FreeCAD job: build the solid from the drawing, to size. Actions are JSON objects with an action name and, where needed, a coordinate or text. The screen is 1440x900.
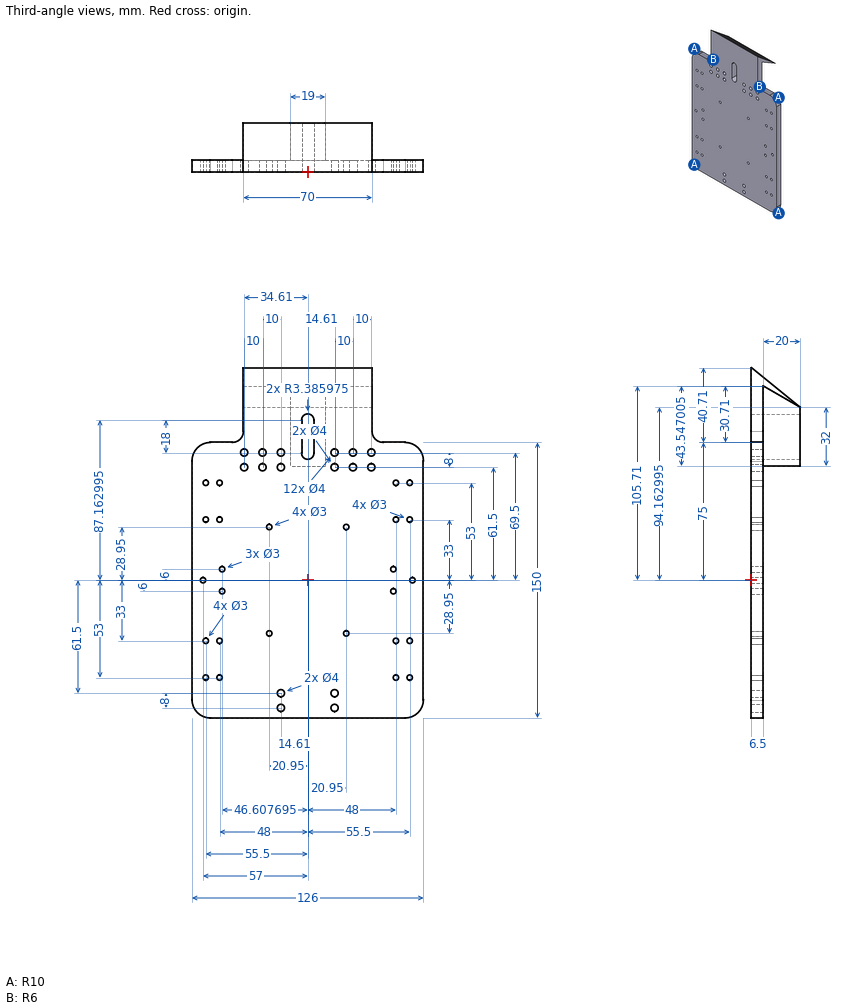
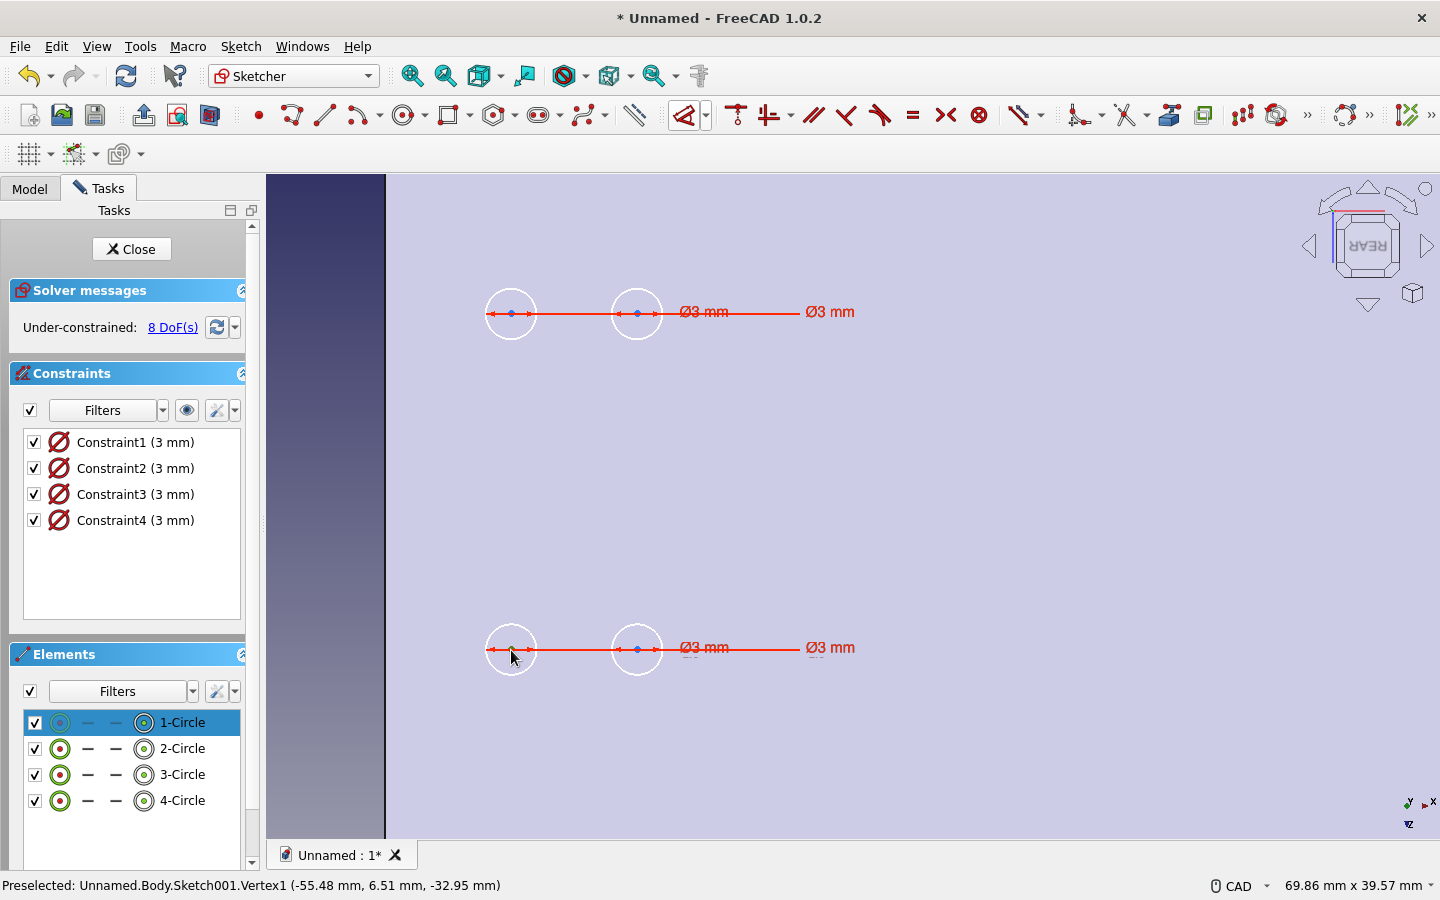
{"action": "left_click", "coordinate": [637, 650]}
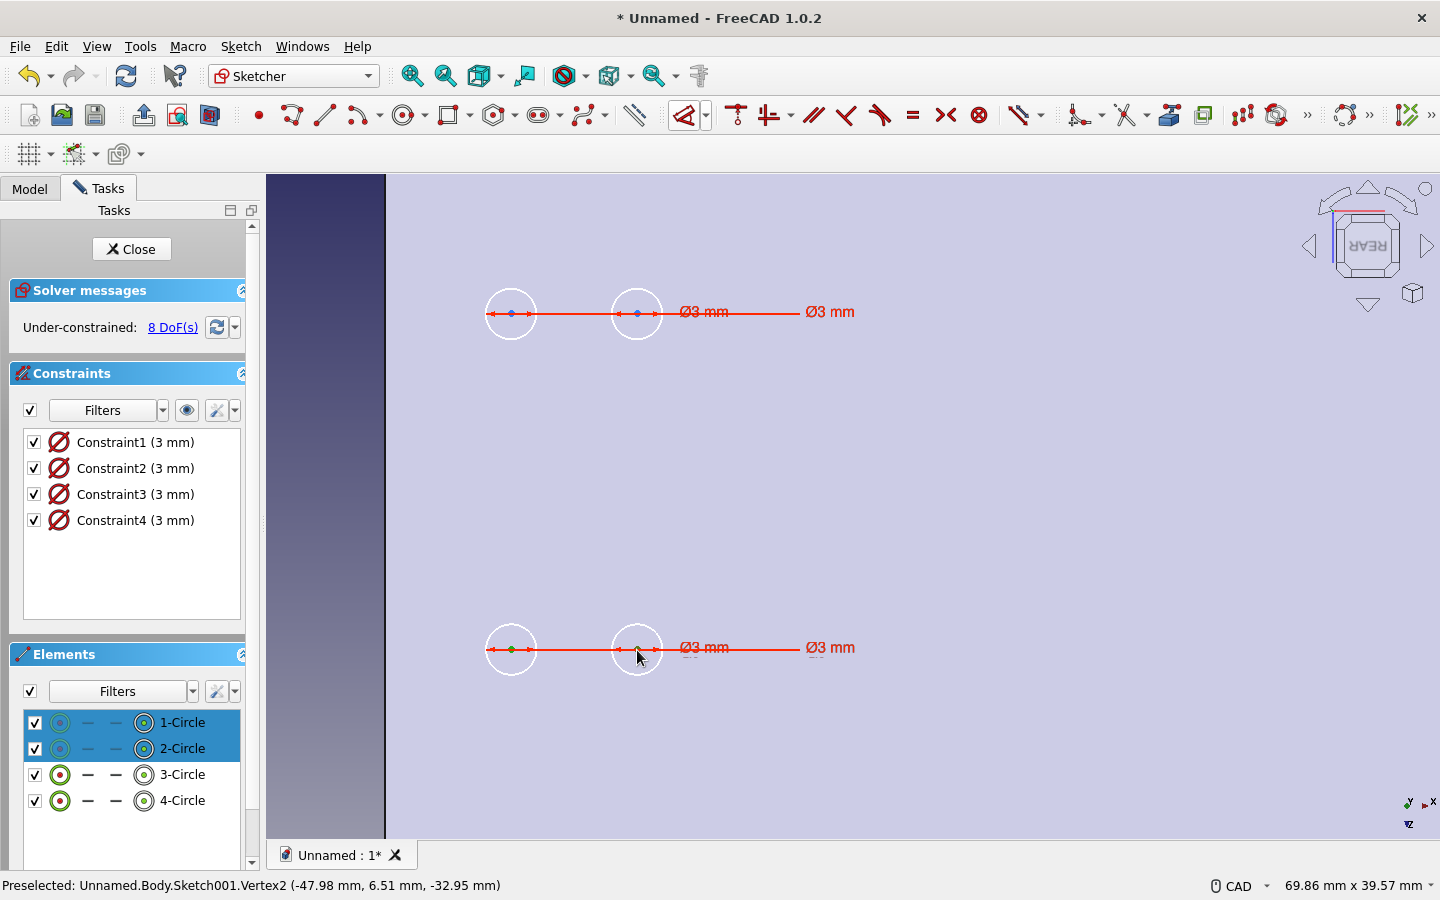
{"action": "left_click", "coordinate": [790, 116]}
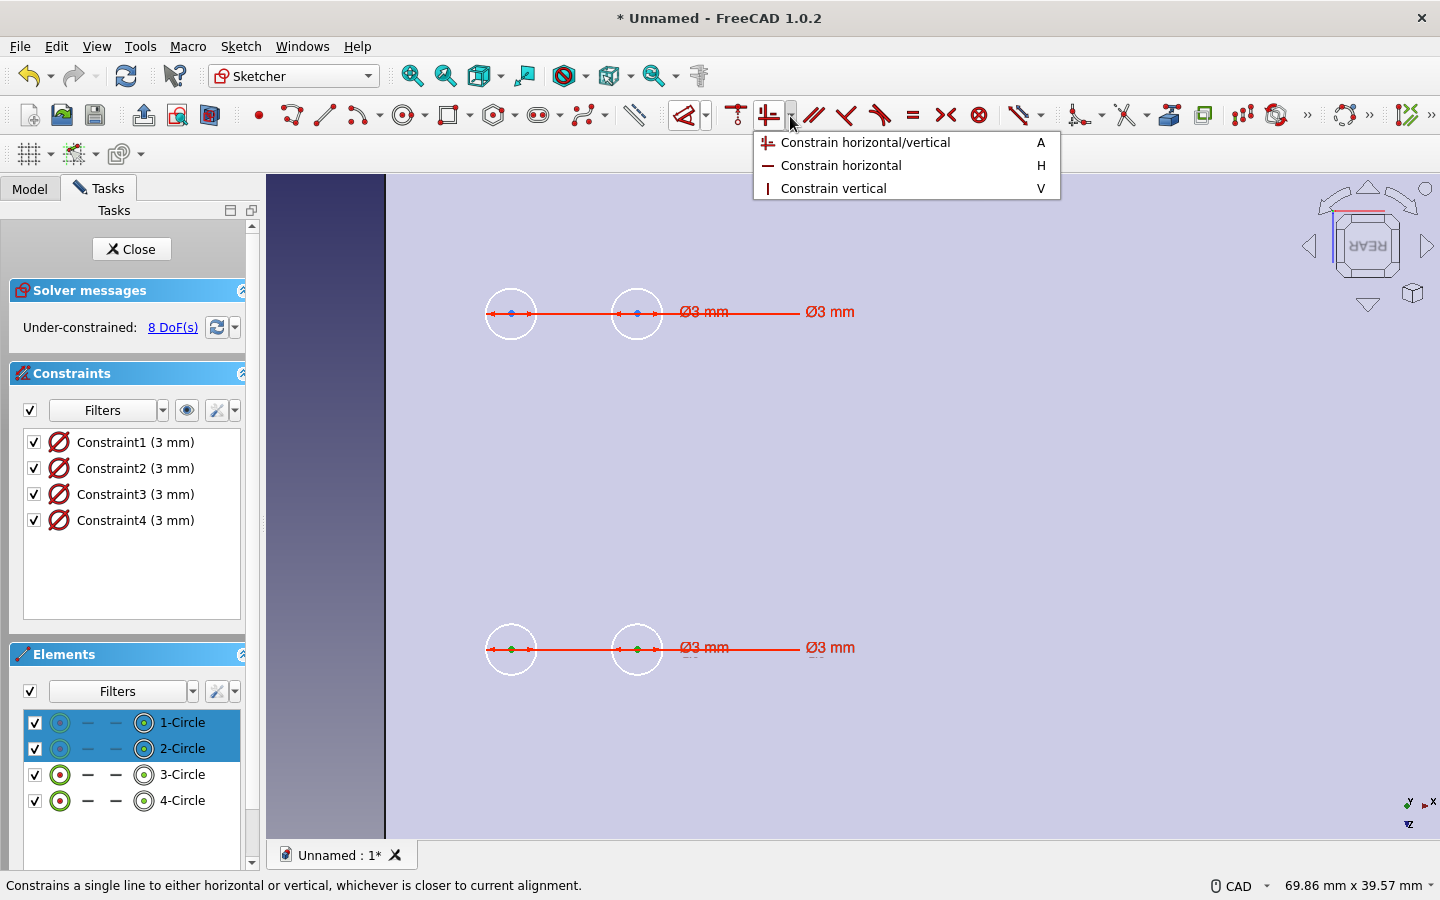
{"action": "left_click", "coordinate": [907, 166]}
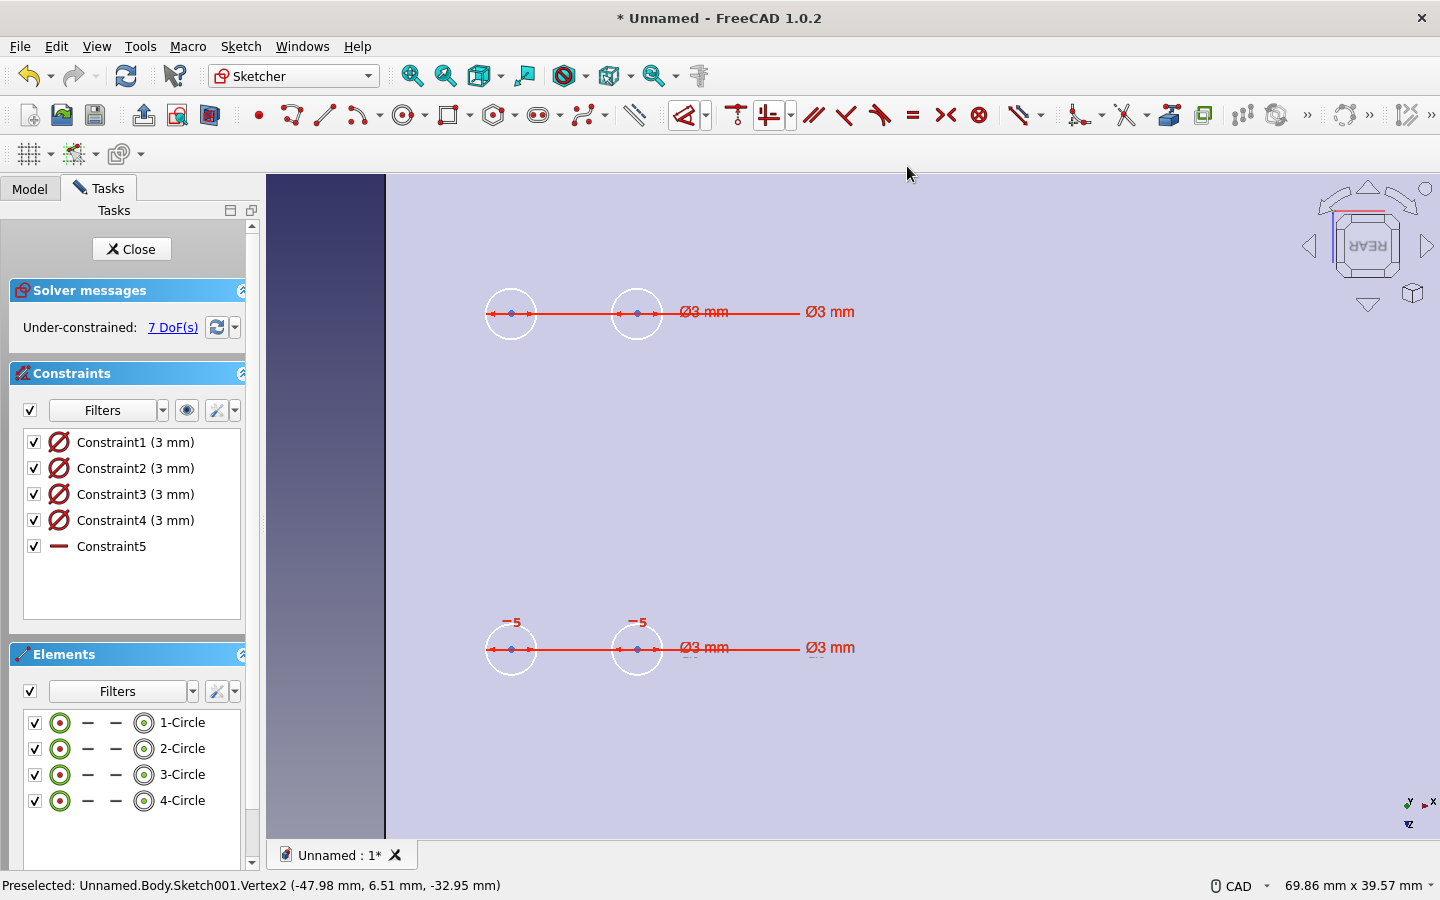
{"action": "left_click", "coordinate": [637, 650]}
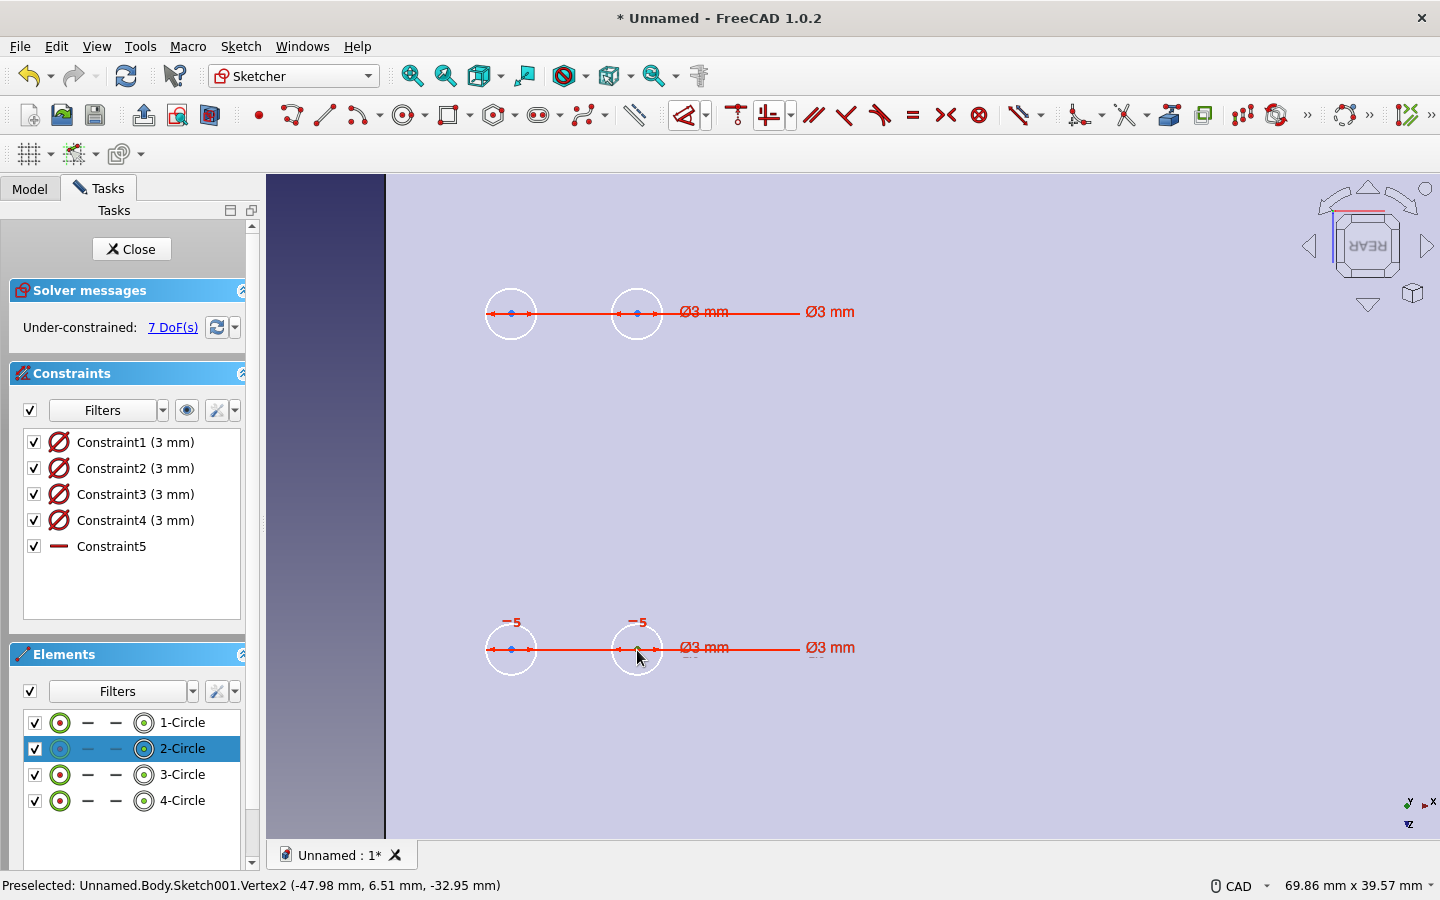
{"action": "left_click", "coordinate": [637, 314]}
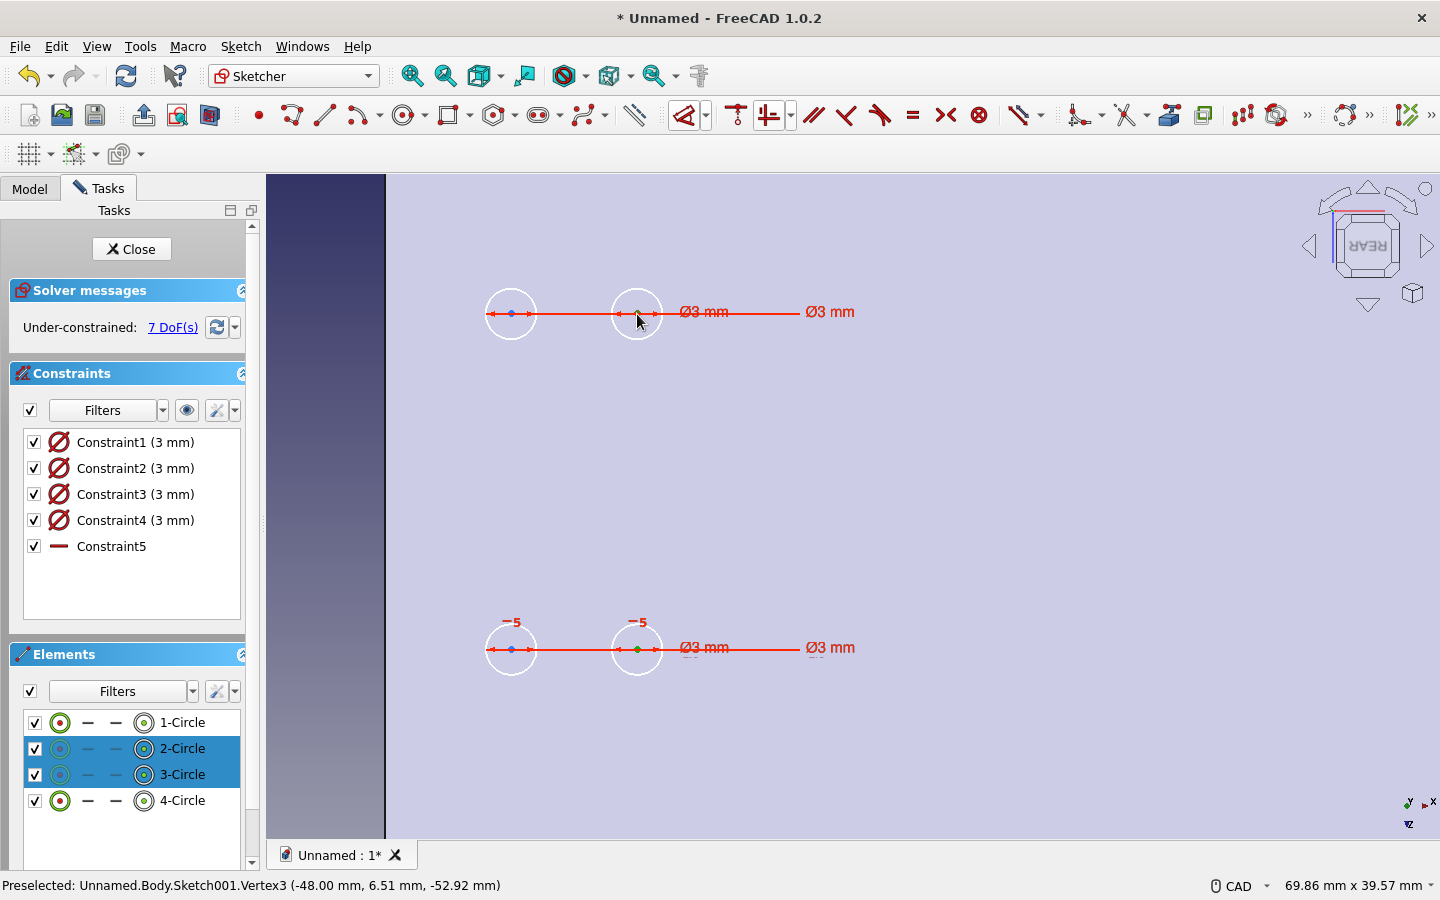
{"action": "key", "text": "v"}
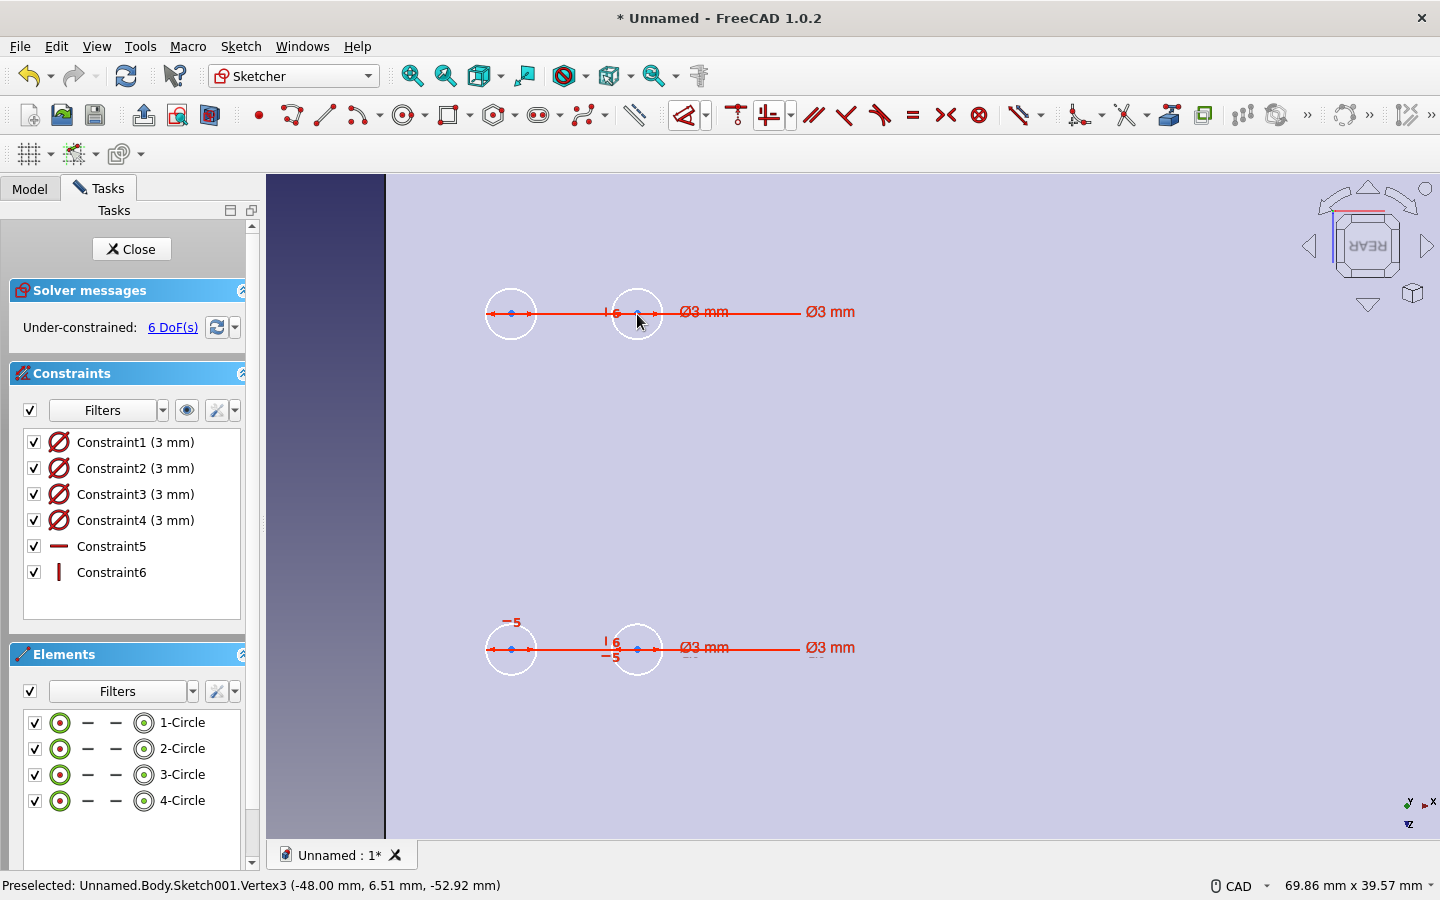
{"action": "left_click", "coordinate": [511, 650]}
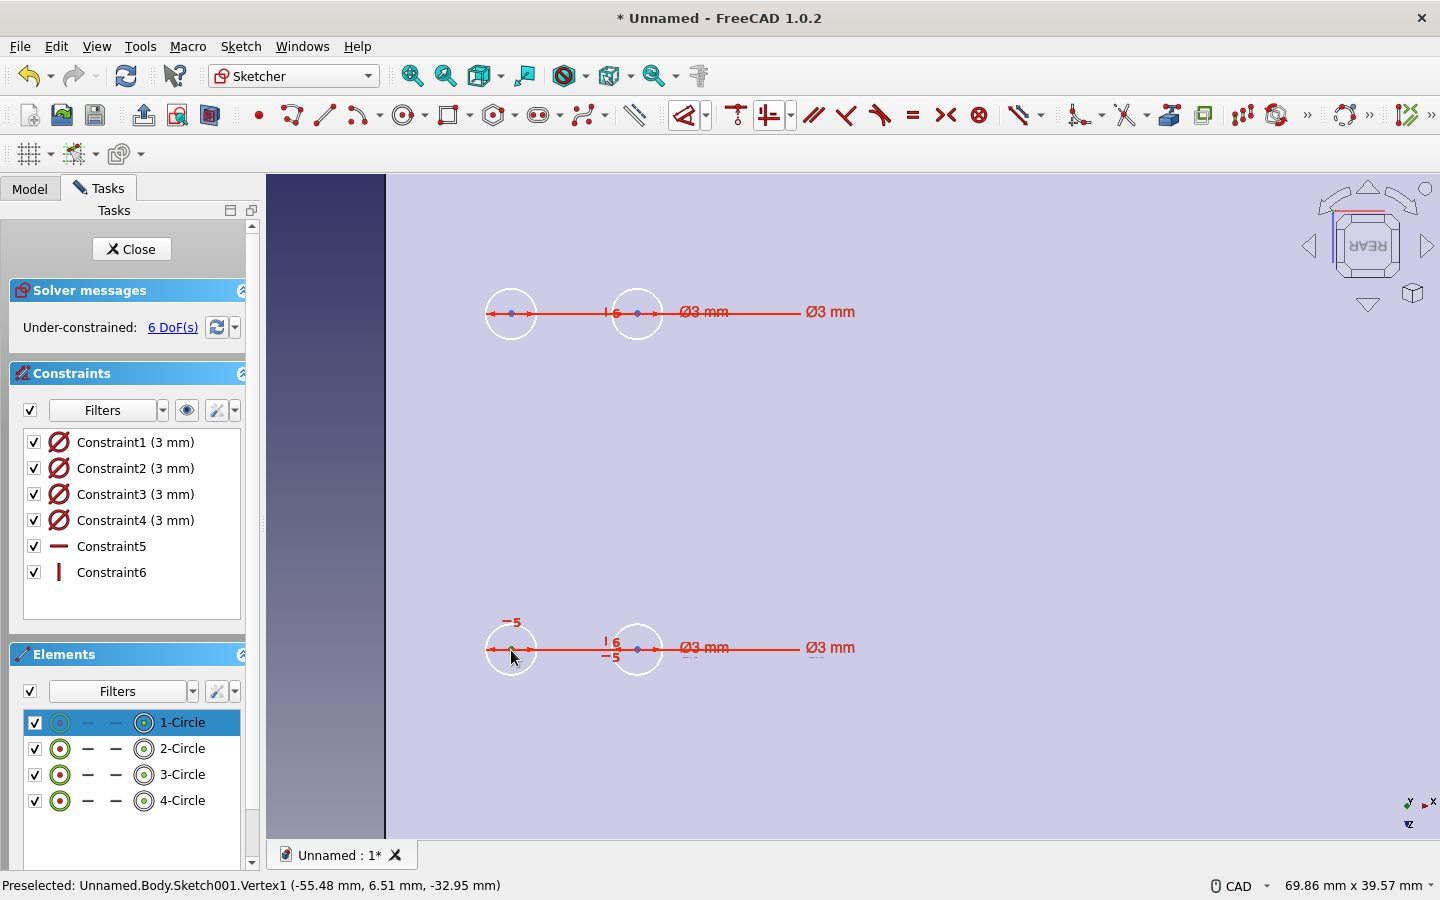
{"action": "left_click", "coordinate": [511, 314]}